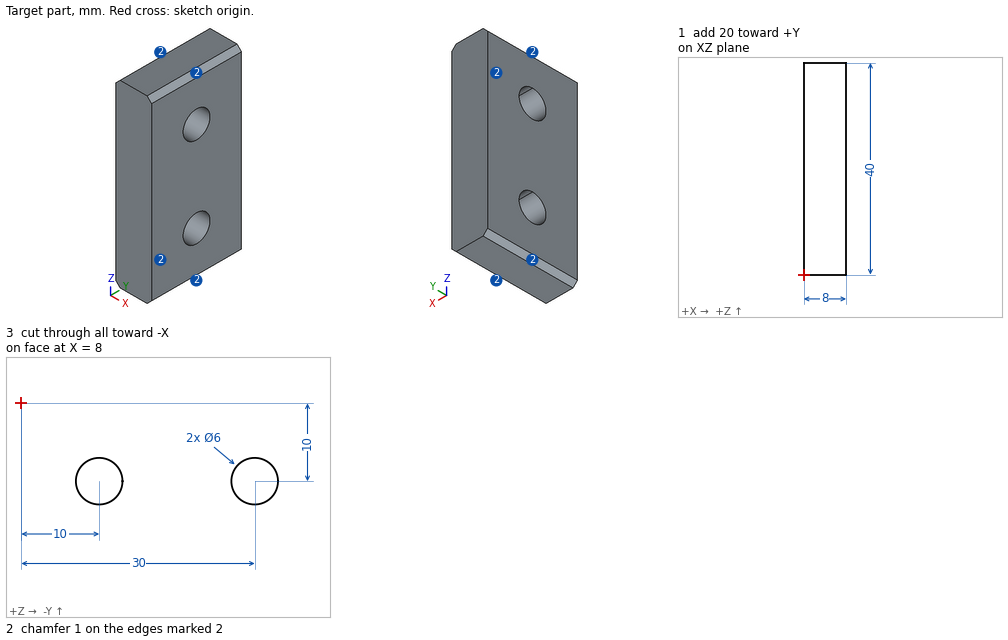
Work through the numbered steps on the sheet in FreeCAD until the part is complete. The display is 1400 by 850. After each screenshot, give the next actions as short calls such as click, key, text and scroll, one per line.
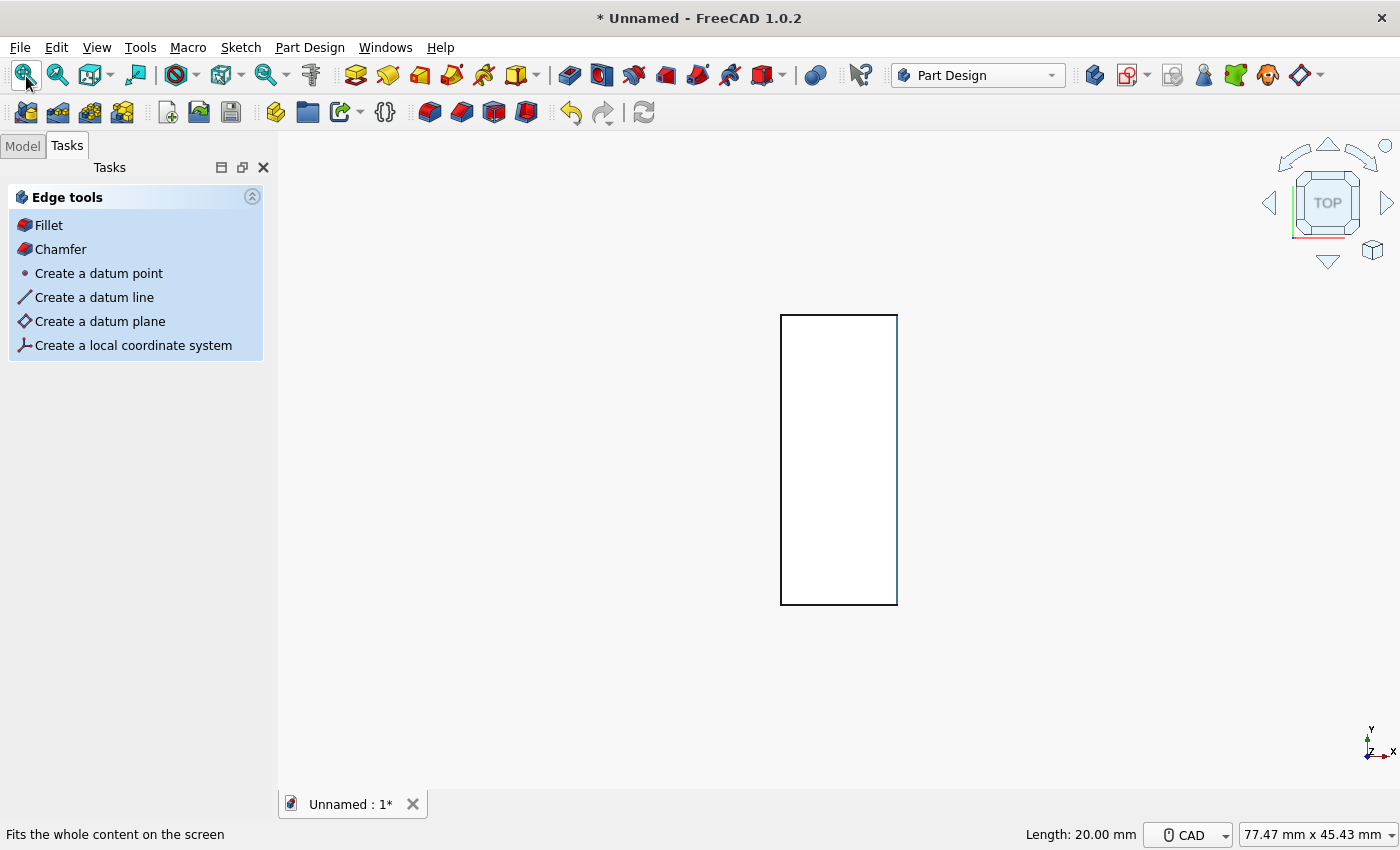
click(781, 459, ctrl)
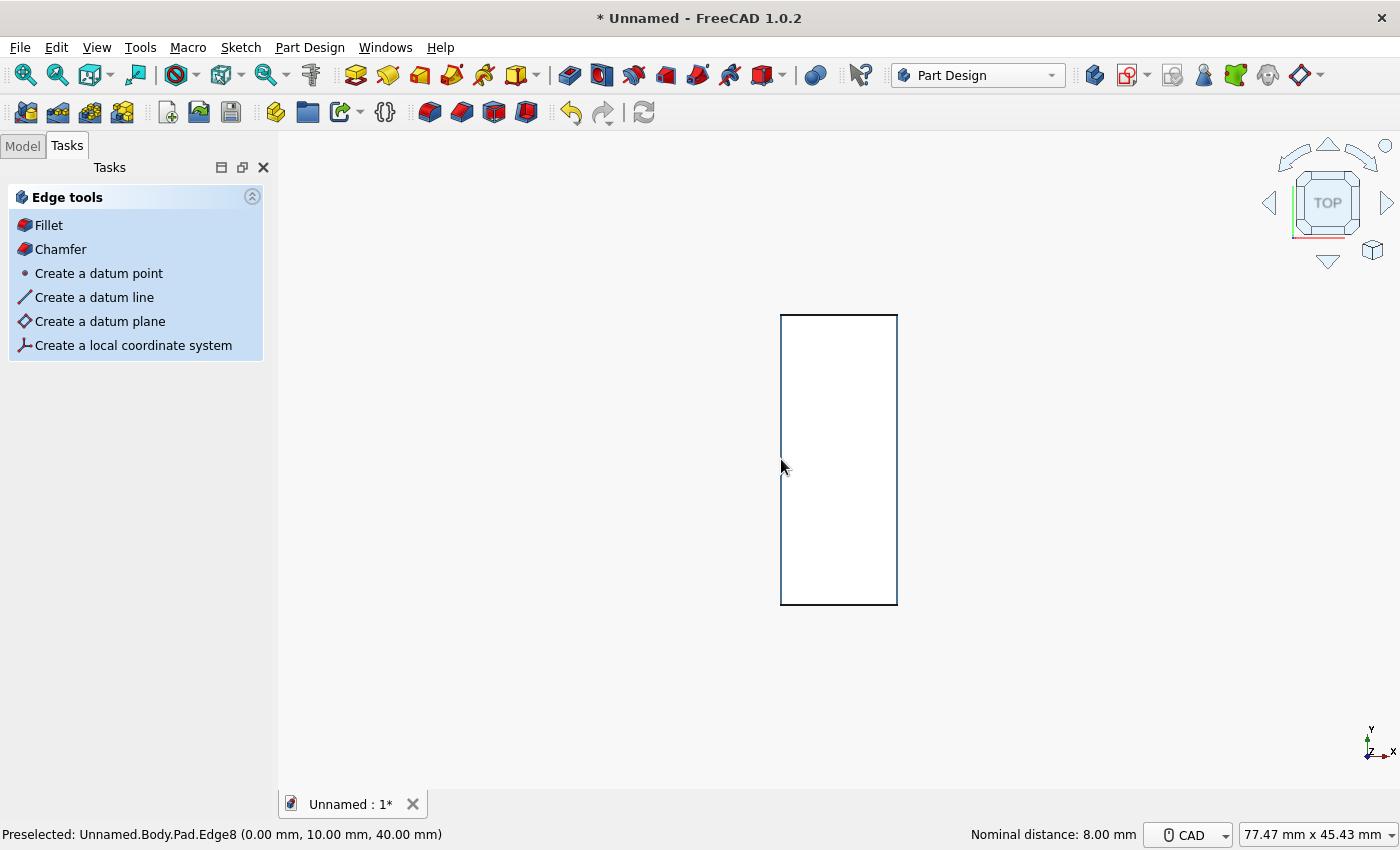
key(1)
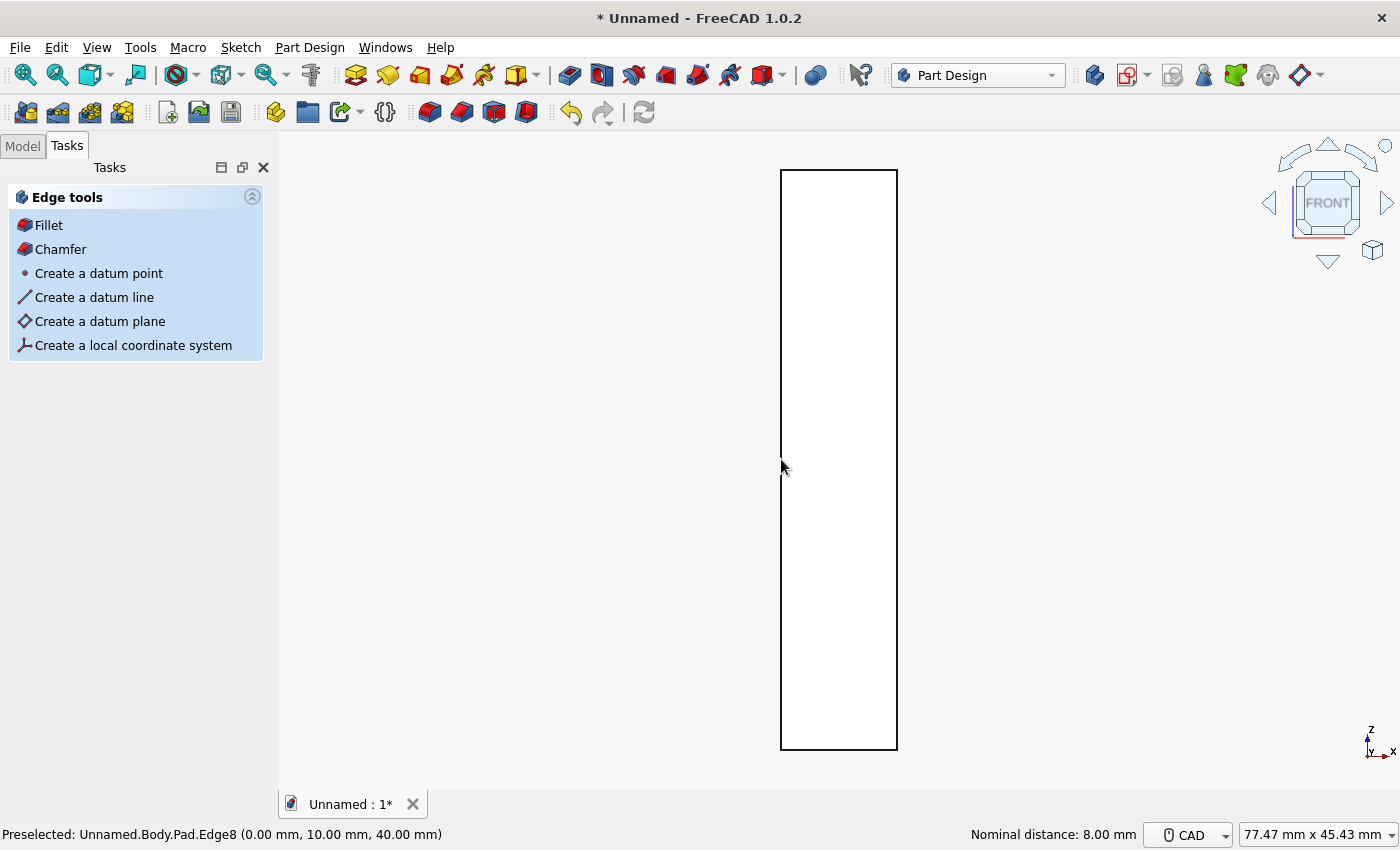
key(3)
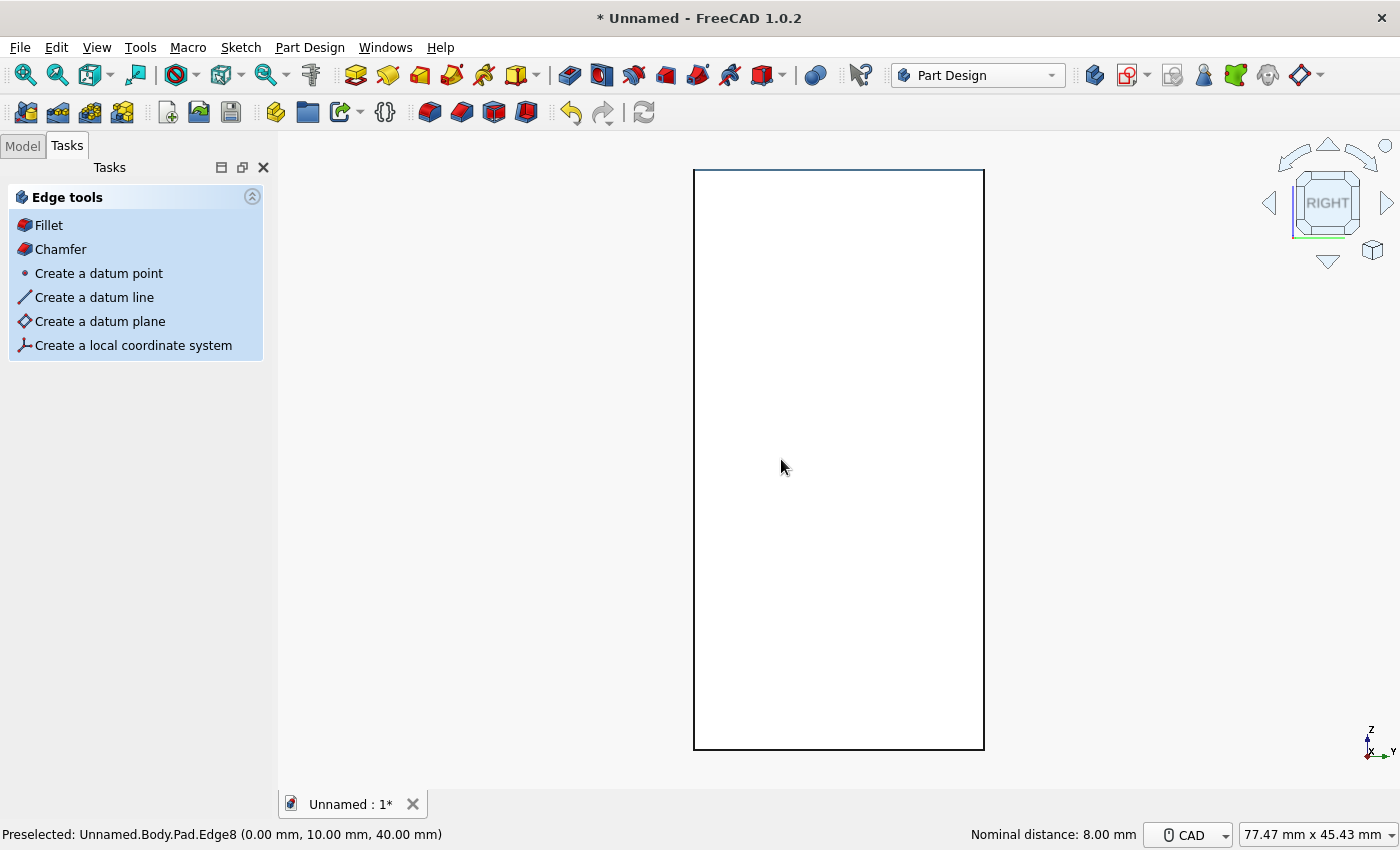
click(839, 749, ctrl)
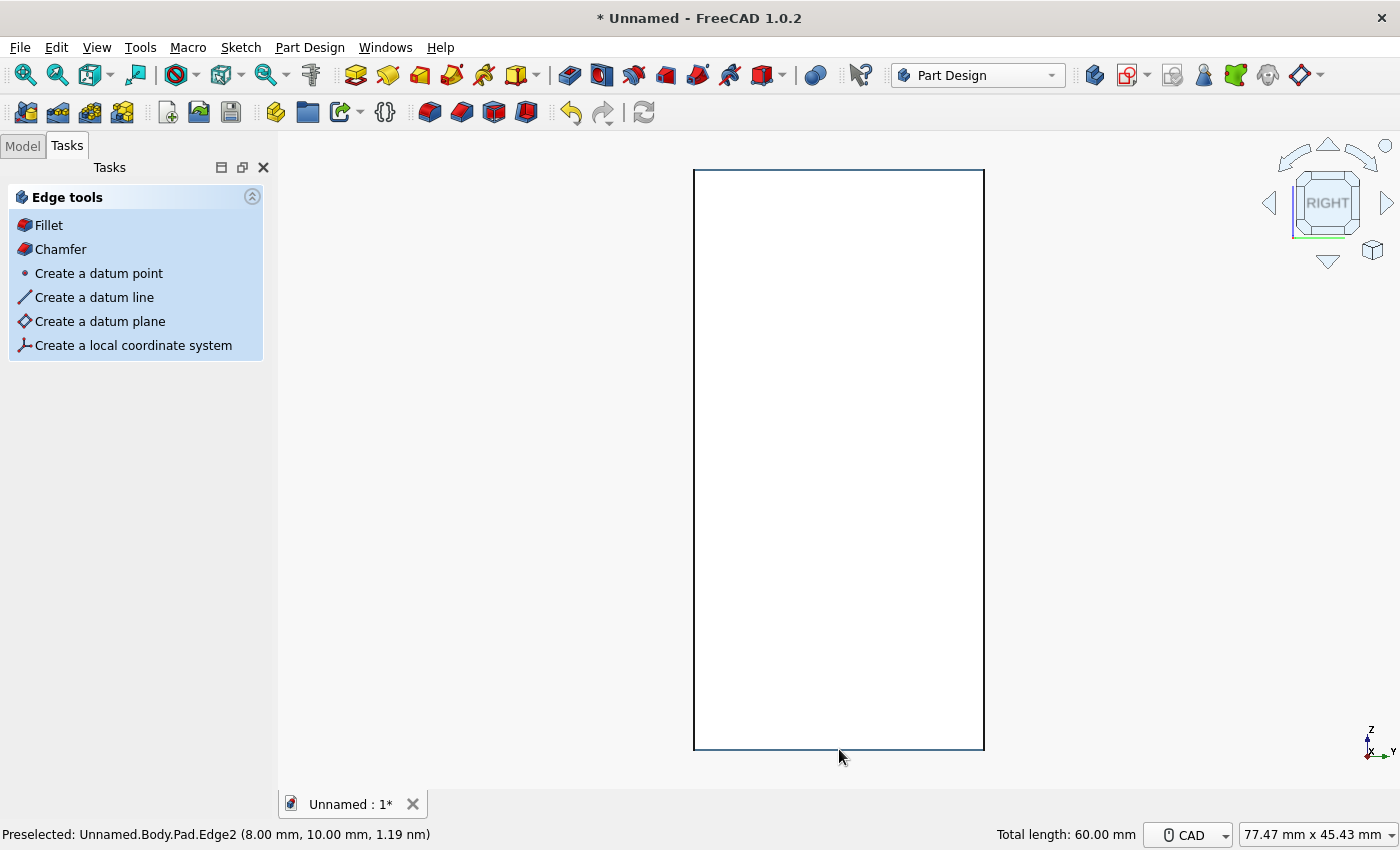
key(5)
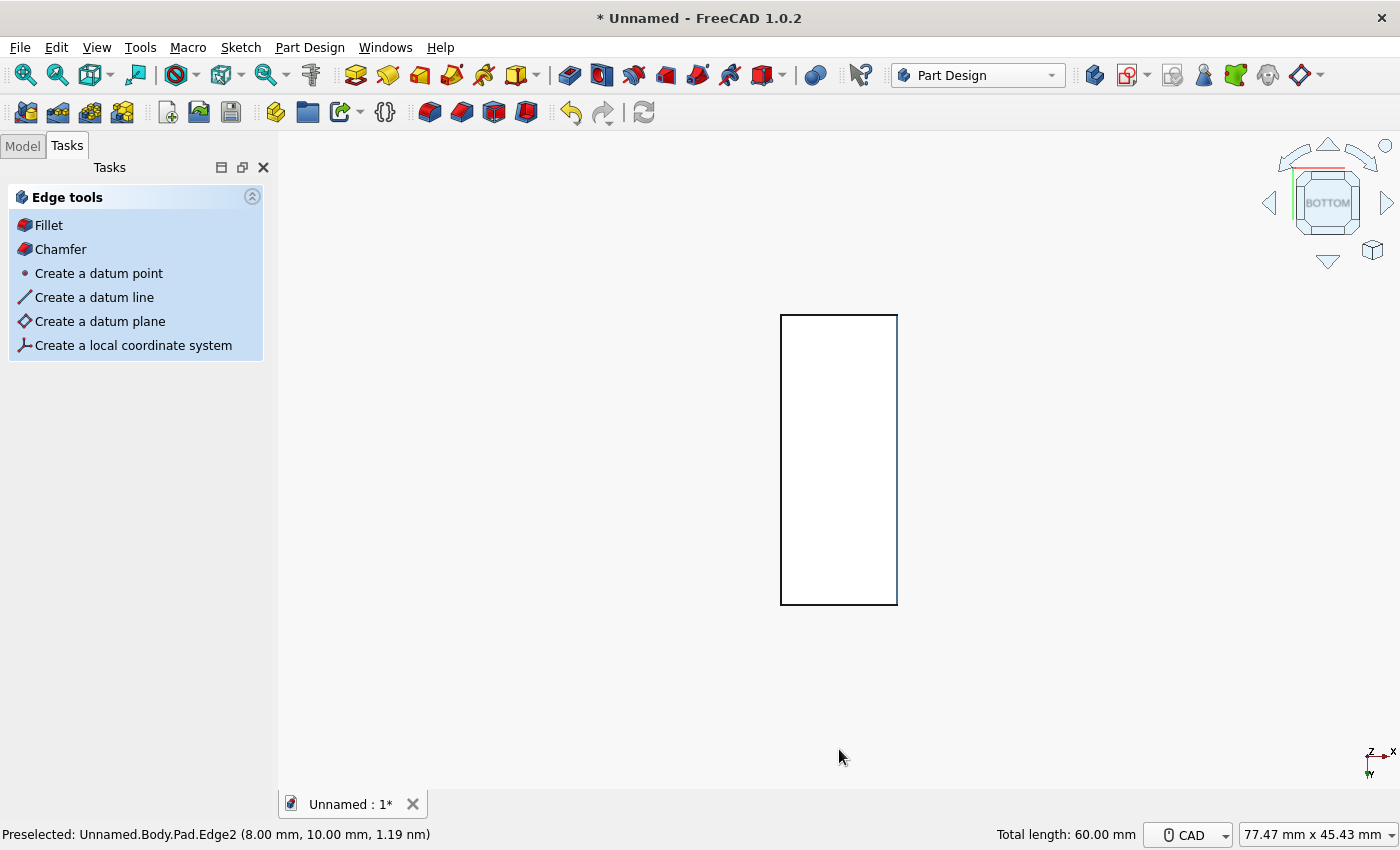
click(26, 76)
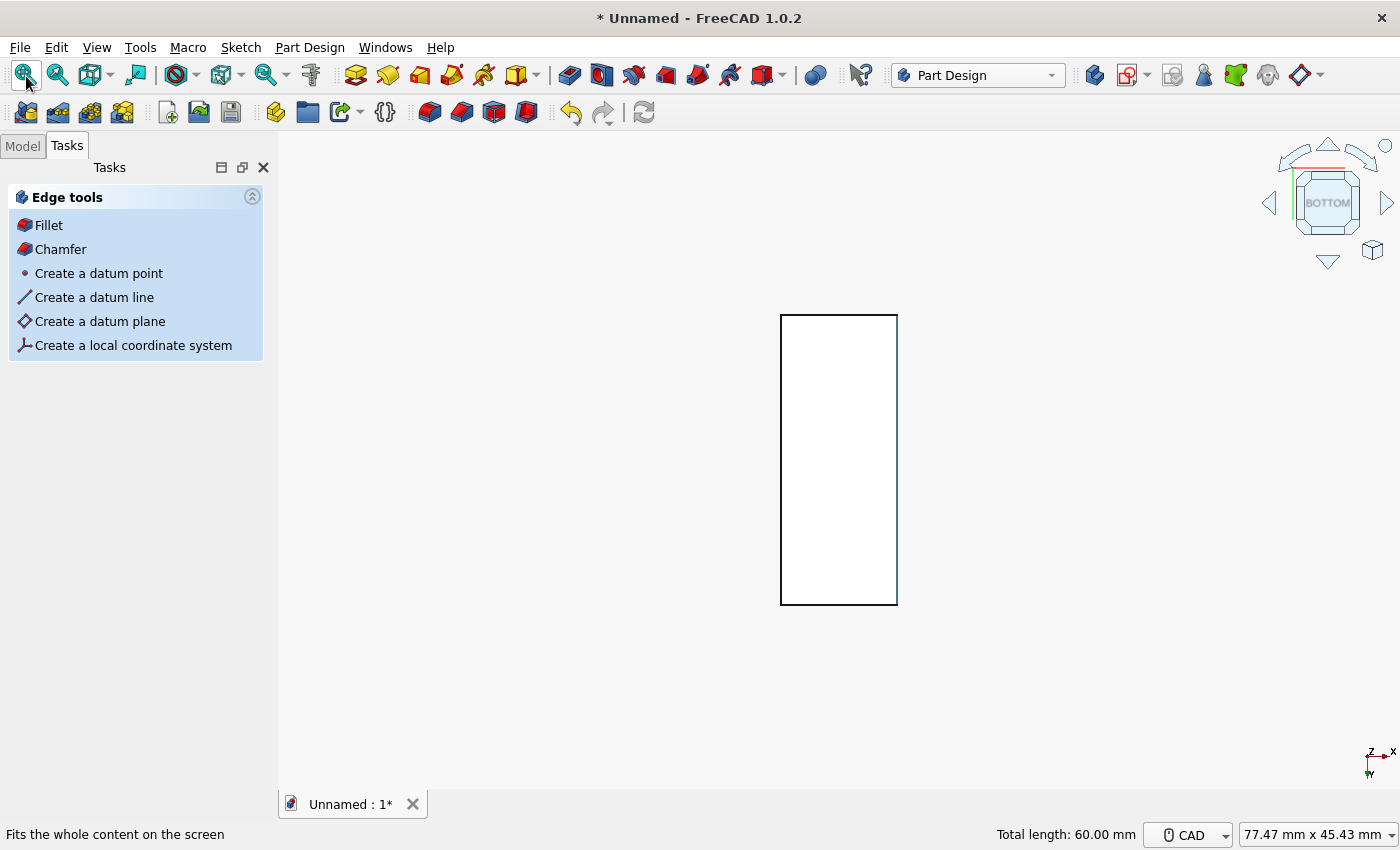
click(781, 488, ctrl)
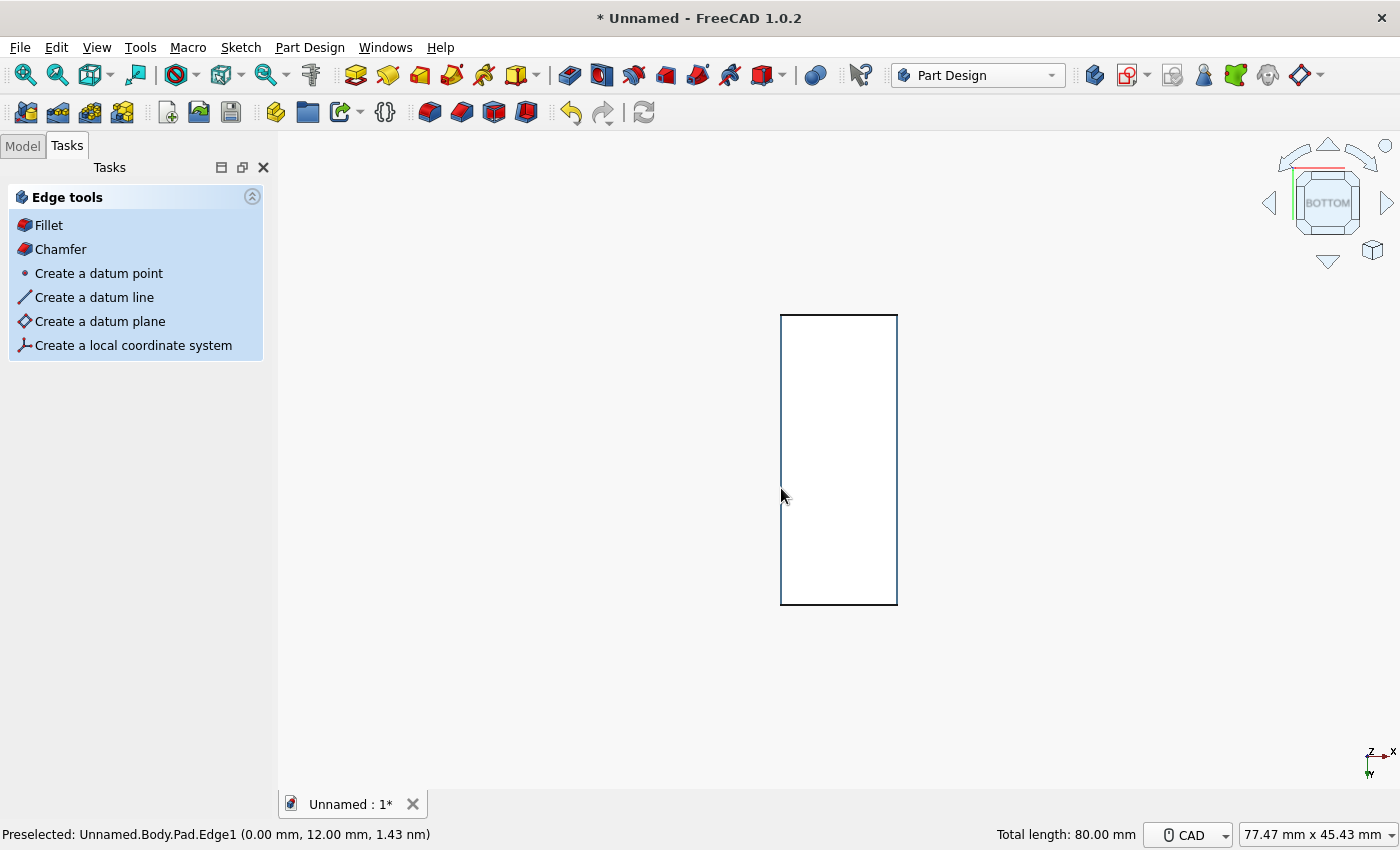
click(462, 112)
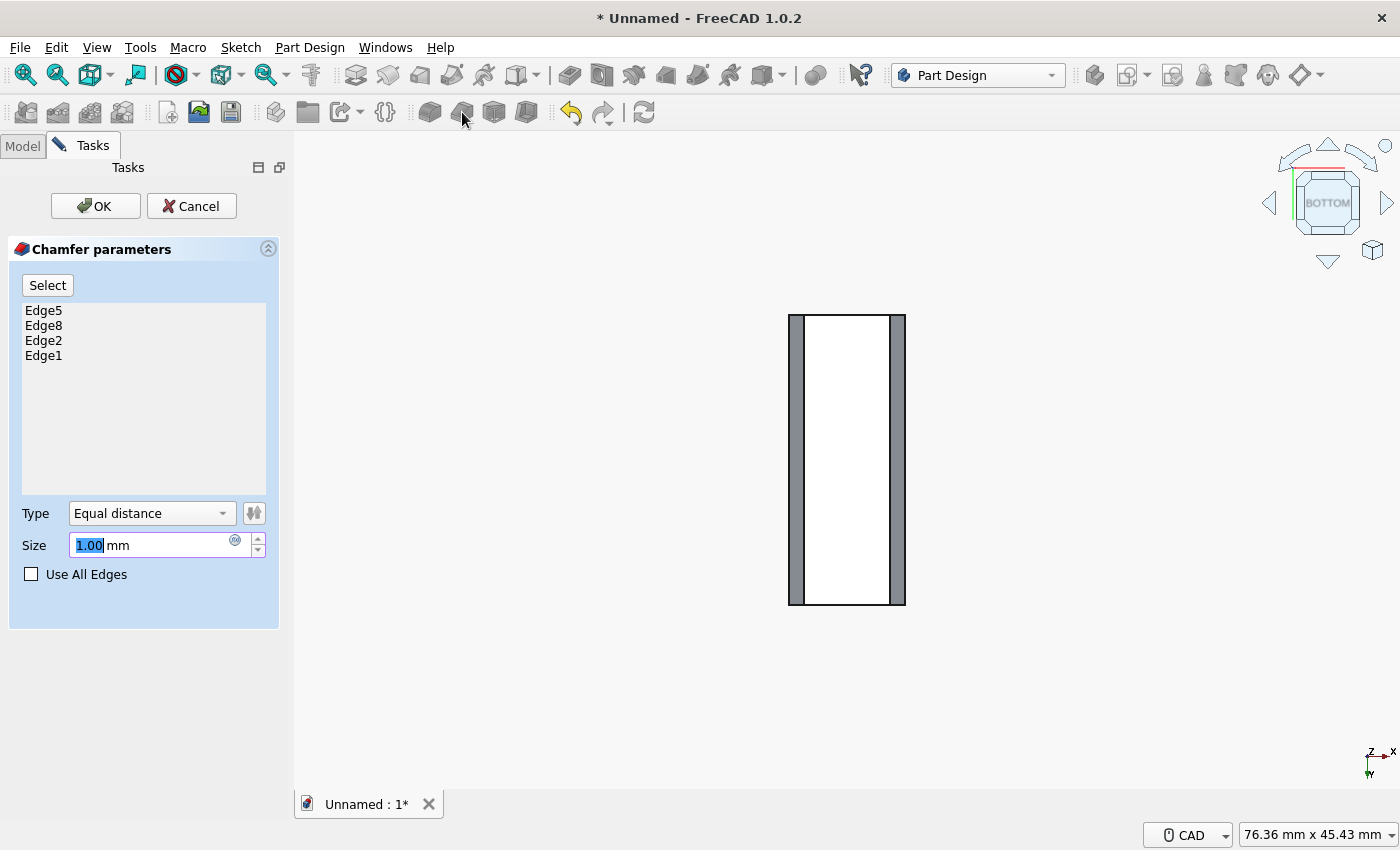
text(1)
key(Tab)